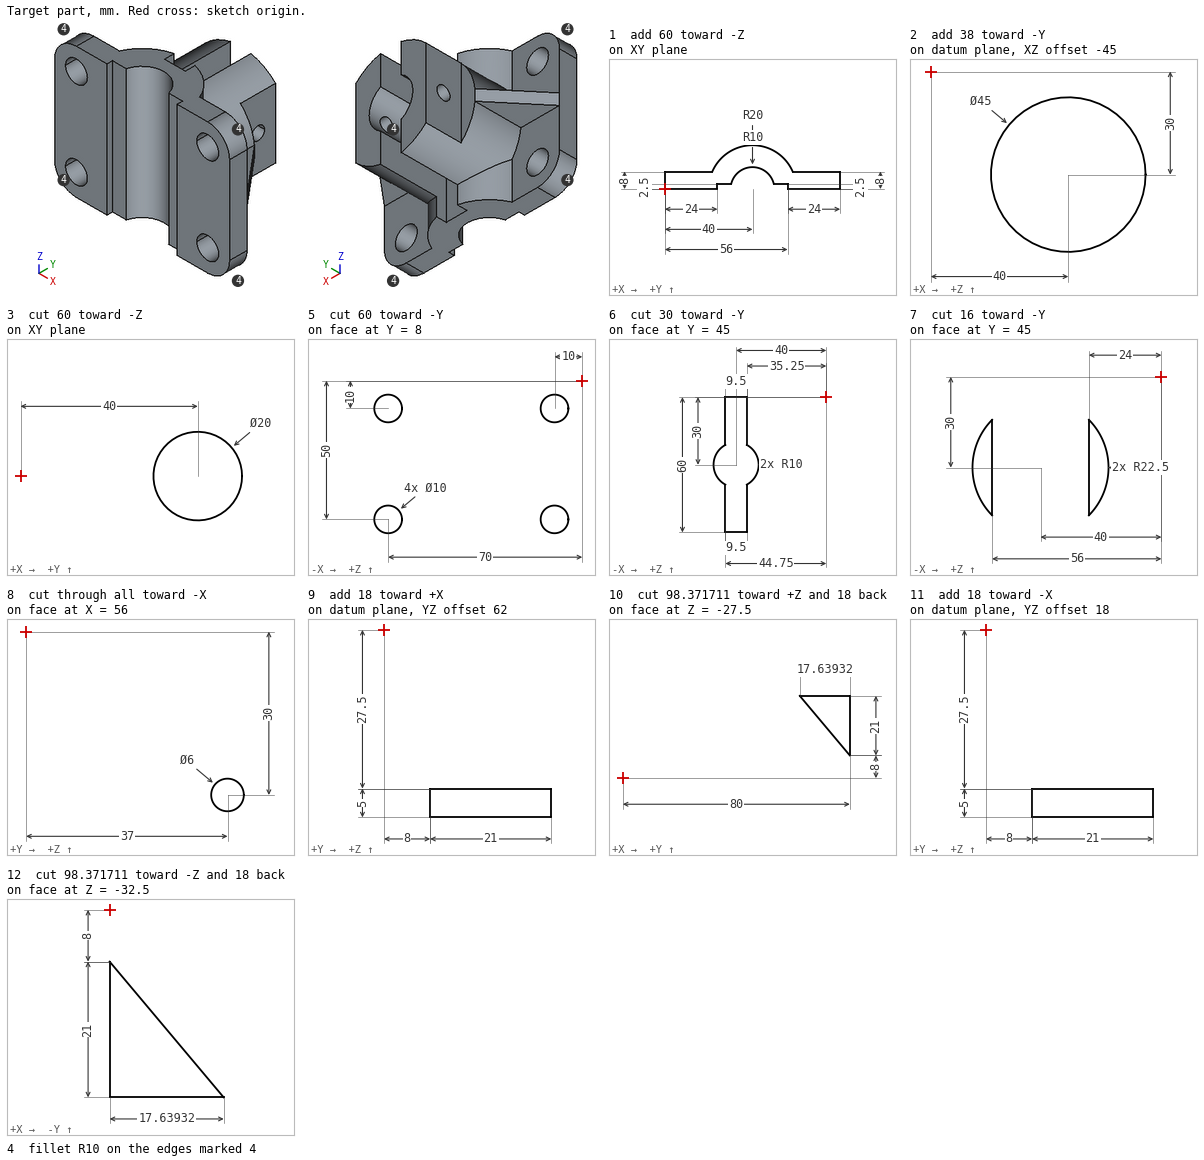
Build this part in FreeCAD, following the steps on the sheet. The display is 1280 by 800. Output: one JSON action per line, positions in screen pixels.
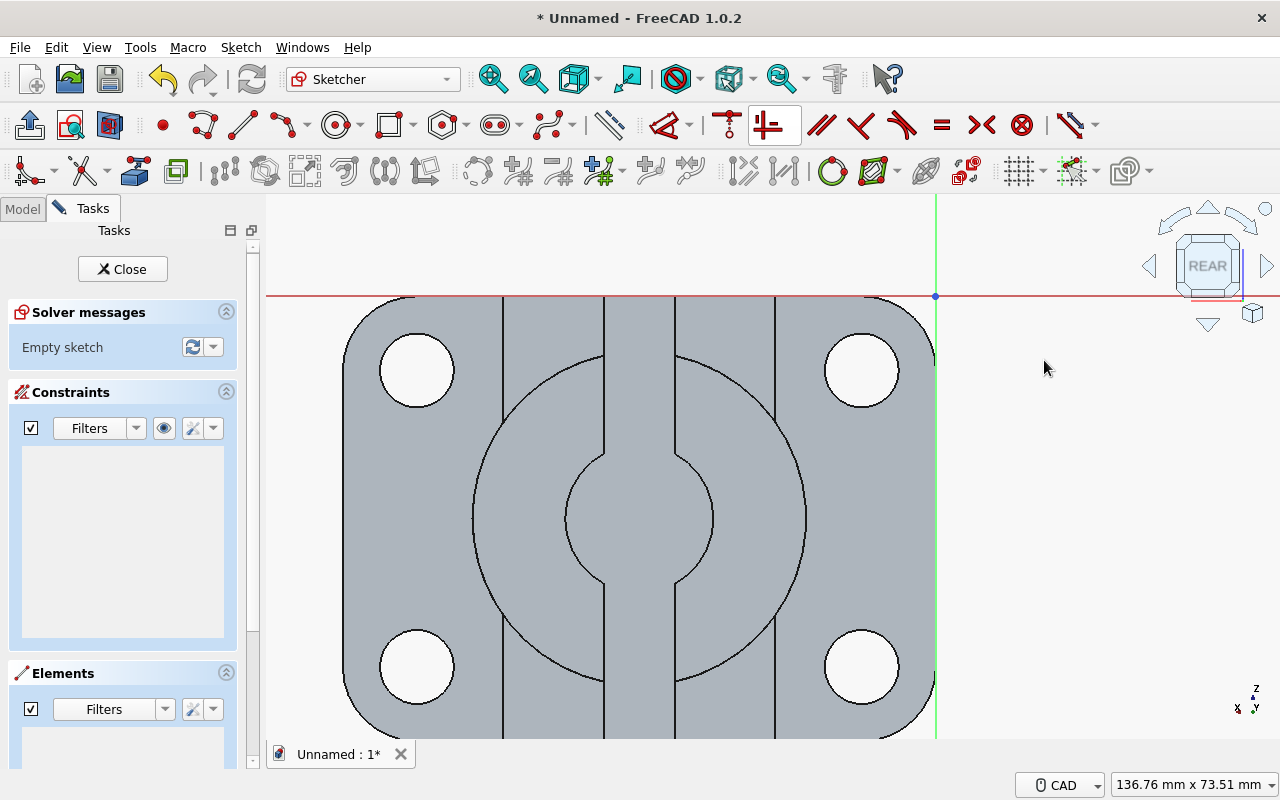
{"action": "left_click", "coordinate": [244, 126]}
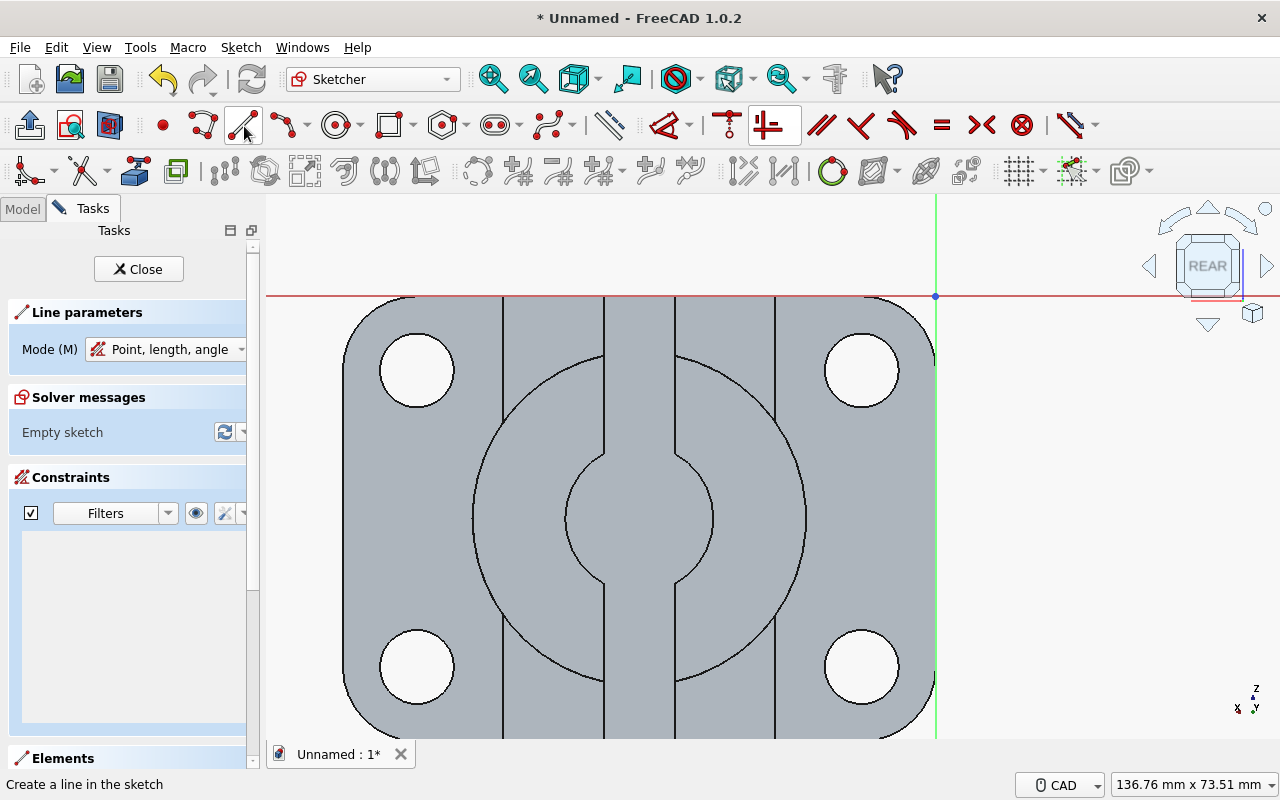
{"action": "left_click", "coordinate": [521, 636]}
{"action": "left_click", "coordinate": [521, 401]}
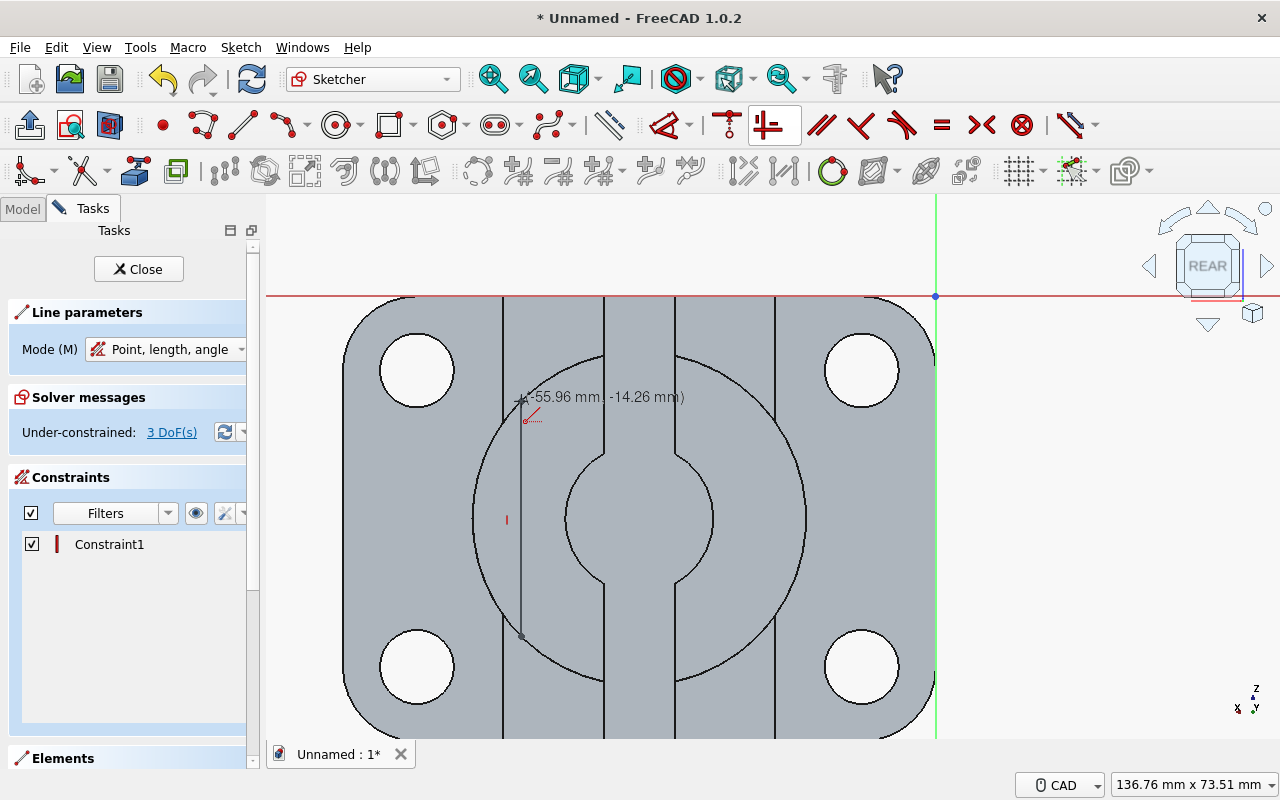
{"action": "left_click", "coordinate": [284, 126]}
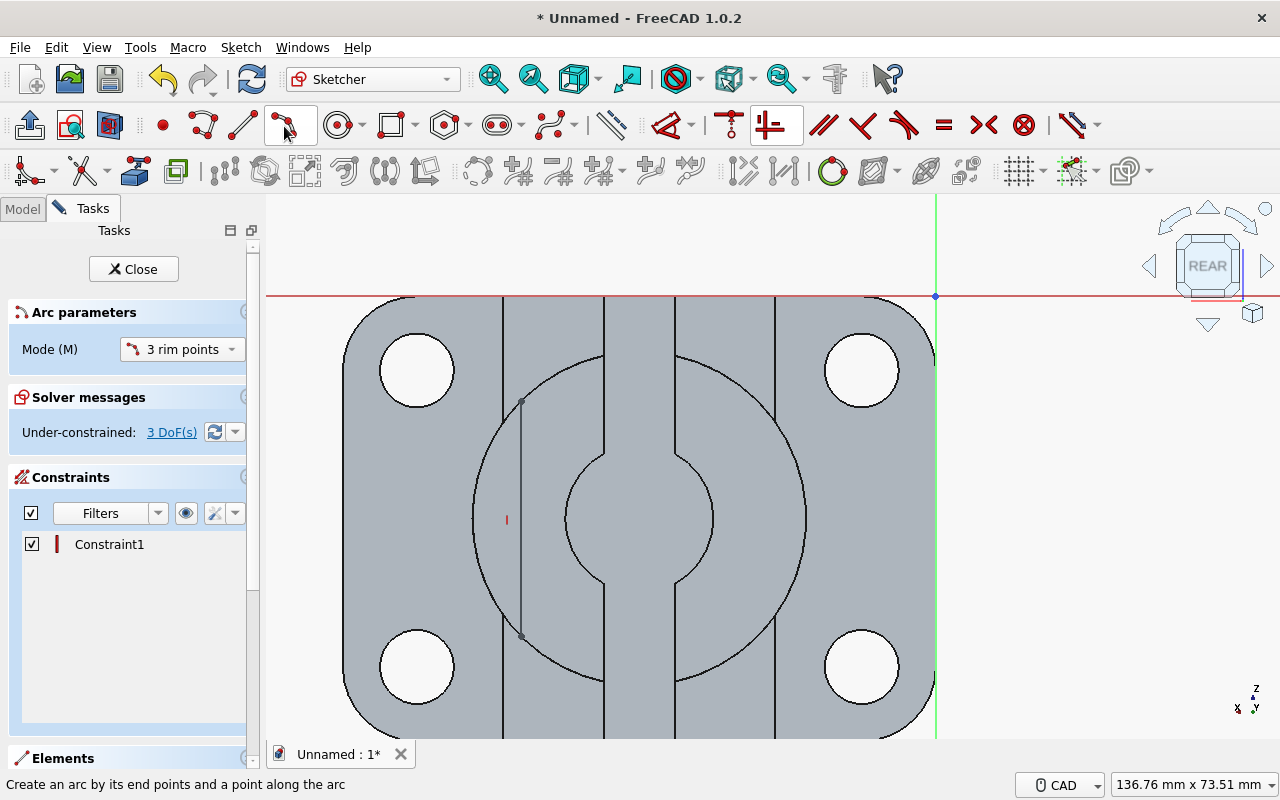
{"action": "left_click", "coordinate": [521, 402]}
{"action": "left_click", "coordinate": [521, 637]}
{"action": "left_click", "coordinate": [473, 519]}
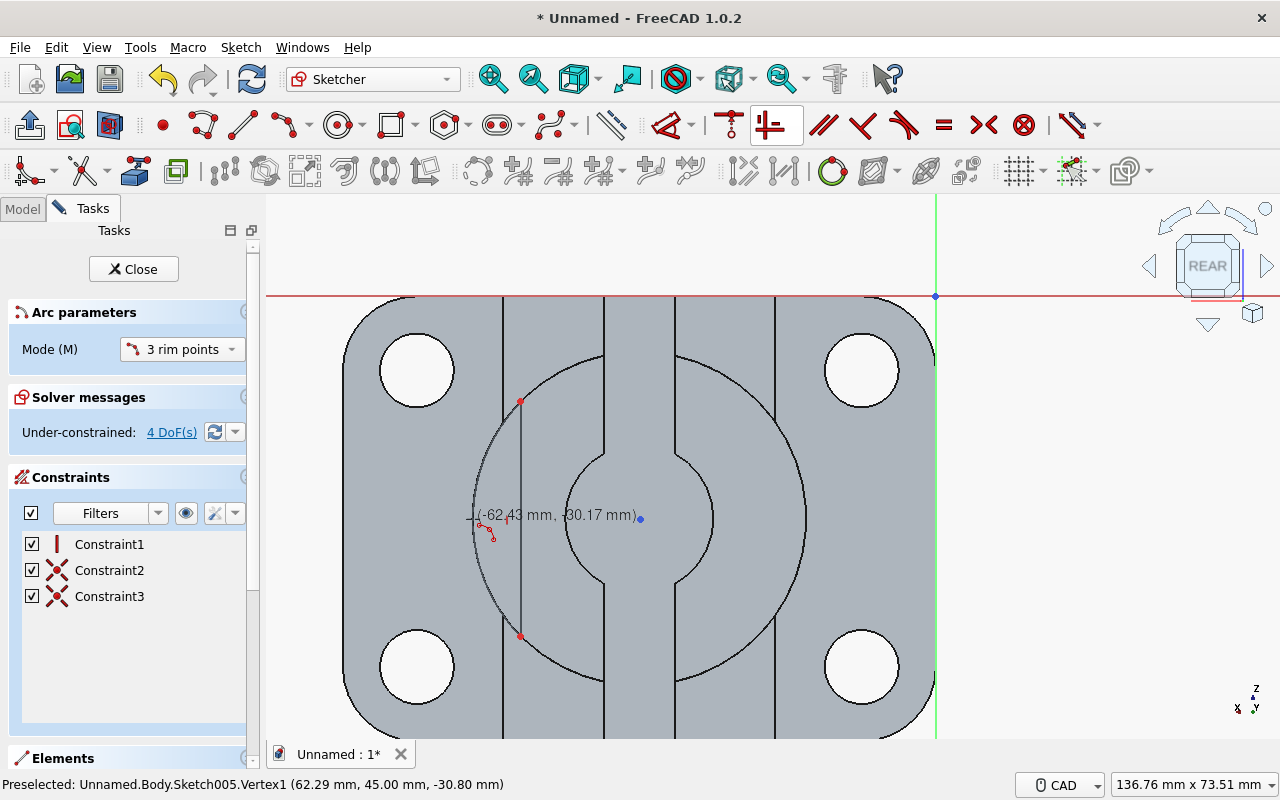
{"action": "left_click", "coordinate": [244, 126]}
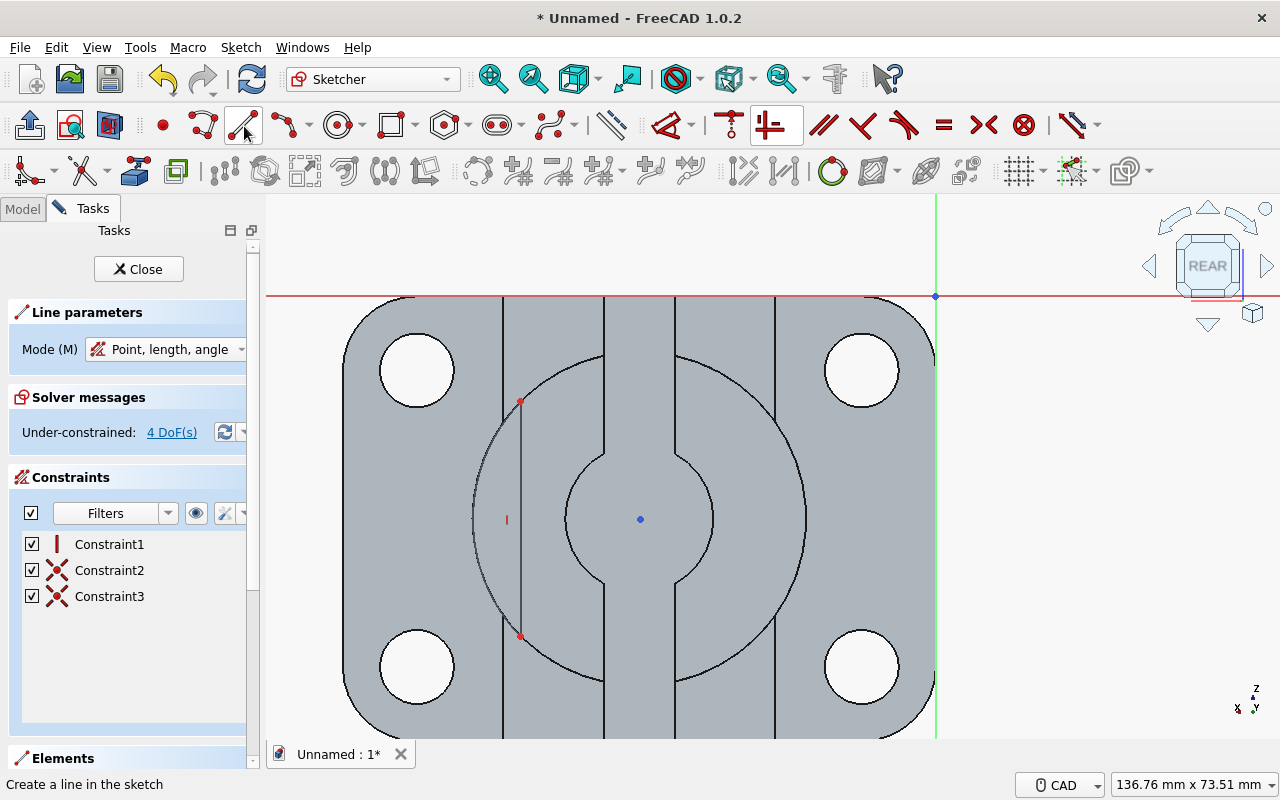
{"action": "left_click", "coordinate": [758, 401]}
{"action": "left_click", "coordinate": [758, 636]}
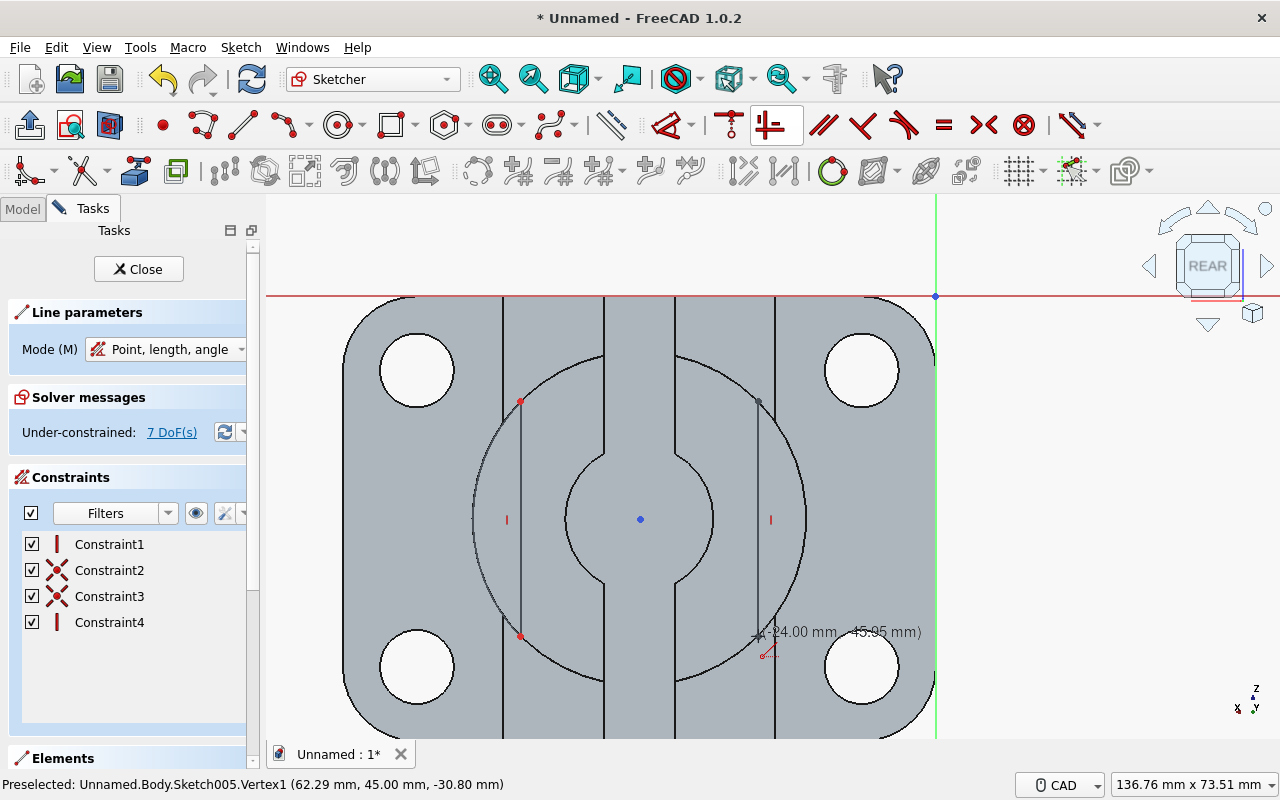
{"action": "left_click", "coordinate": [284, 126]}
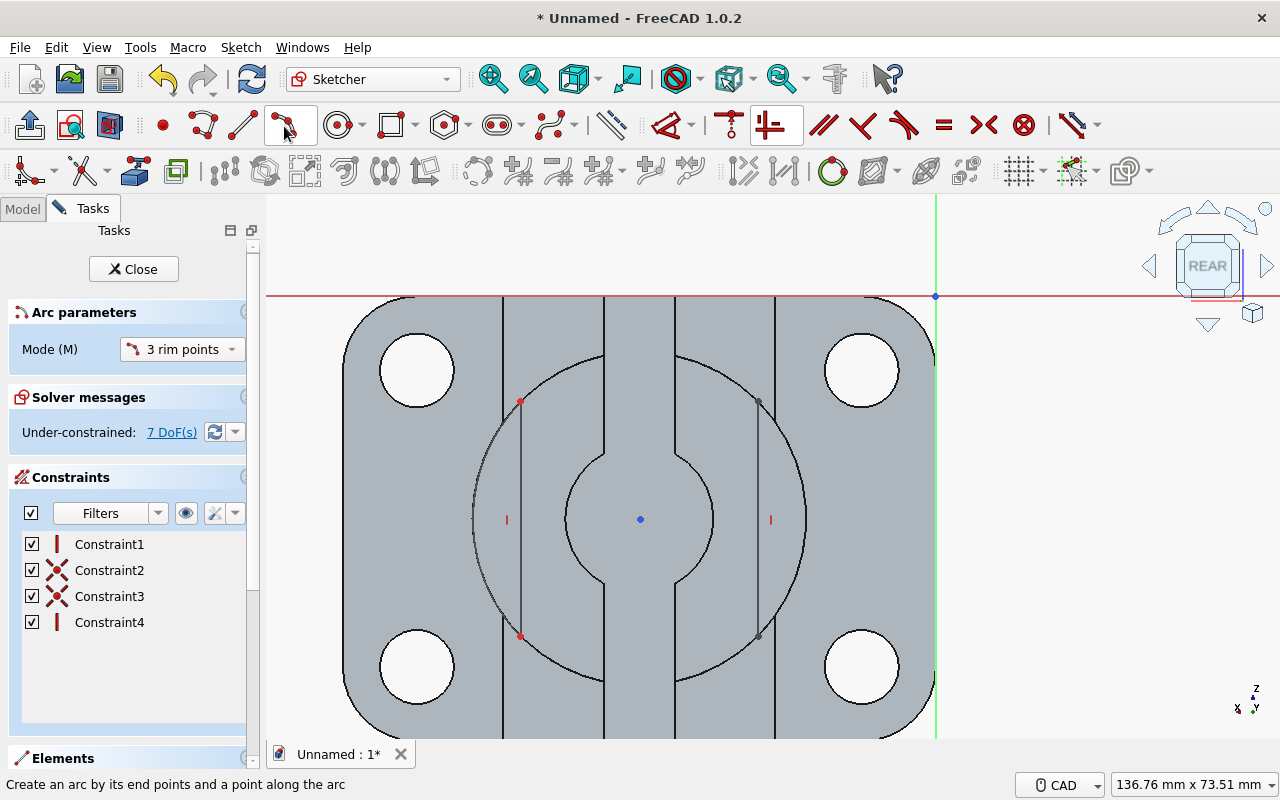
{"action": "left_click", "coordinate": [758, 637]}
{"action": "left_click", "coordinate": [758, 402]}
{"action": "left_click", "coordinate": [806, 519]}
{"action": "key", "text": "Escape"}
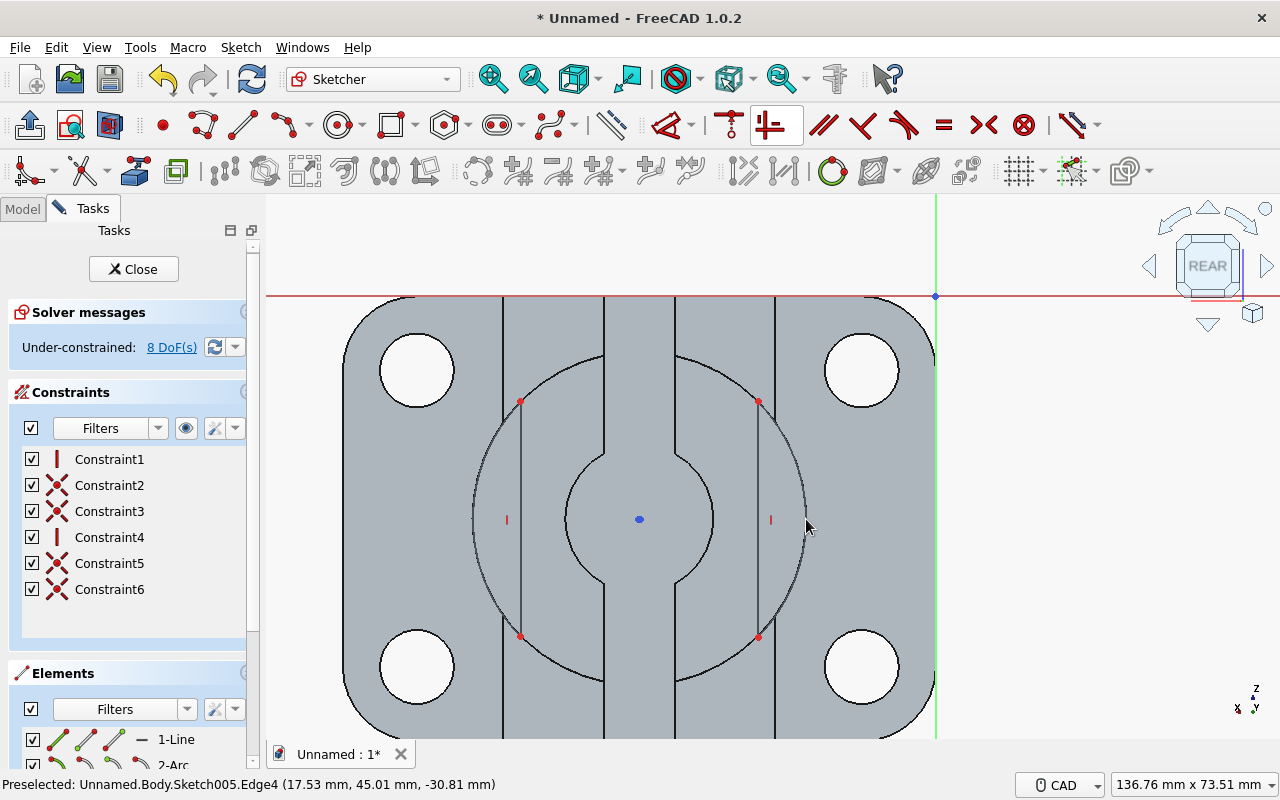
{"action": "left_click", "coordinate": [481, 468]}